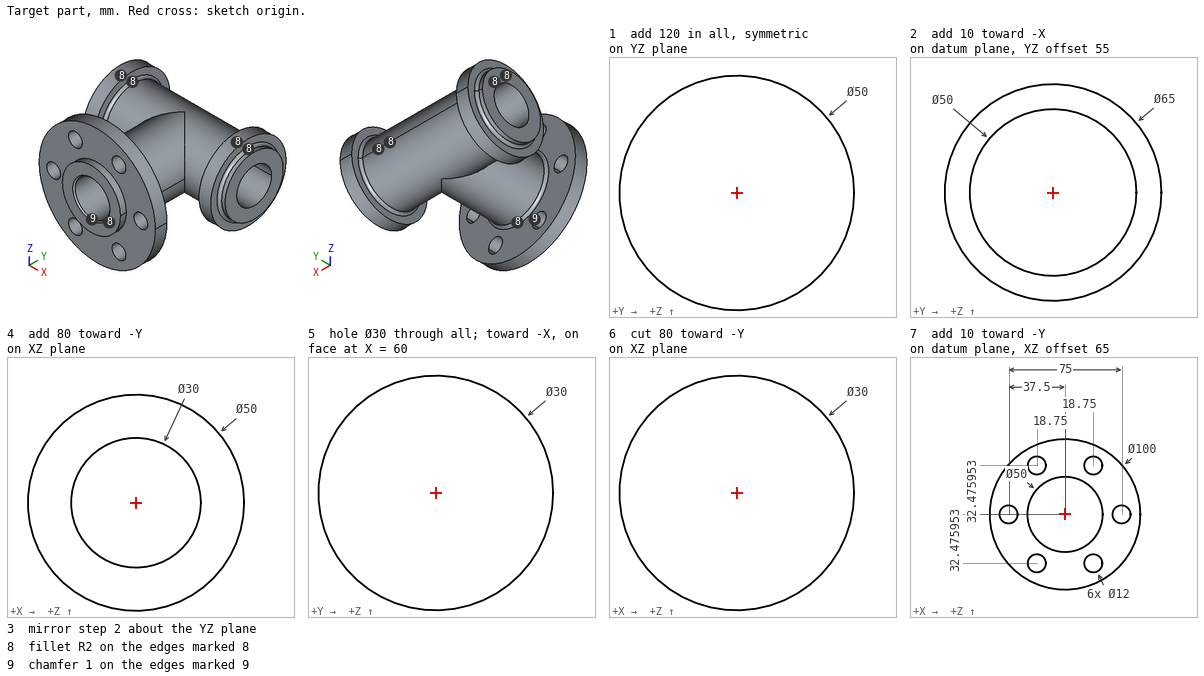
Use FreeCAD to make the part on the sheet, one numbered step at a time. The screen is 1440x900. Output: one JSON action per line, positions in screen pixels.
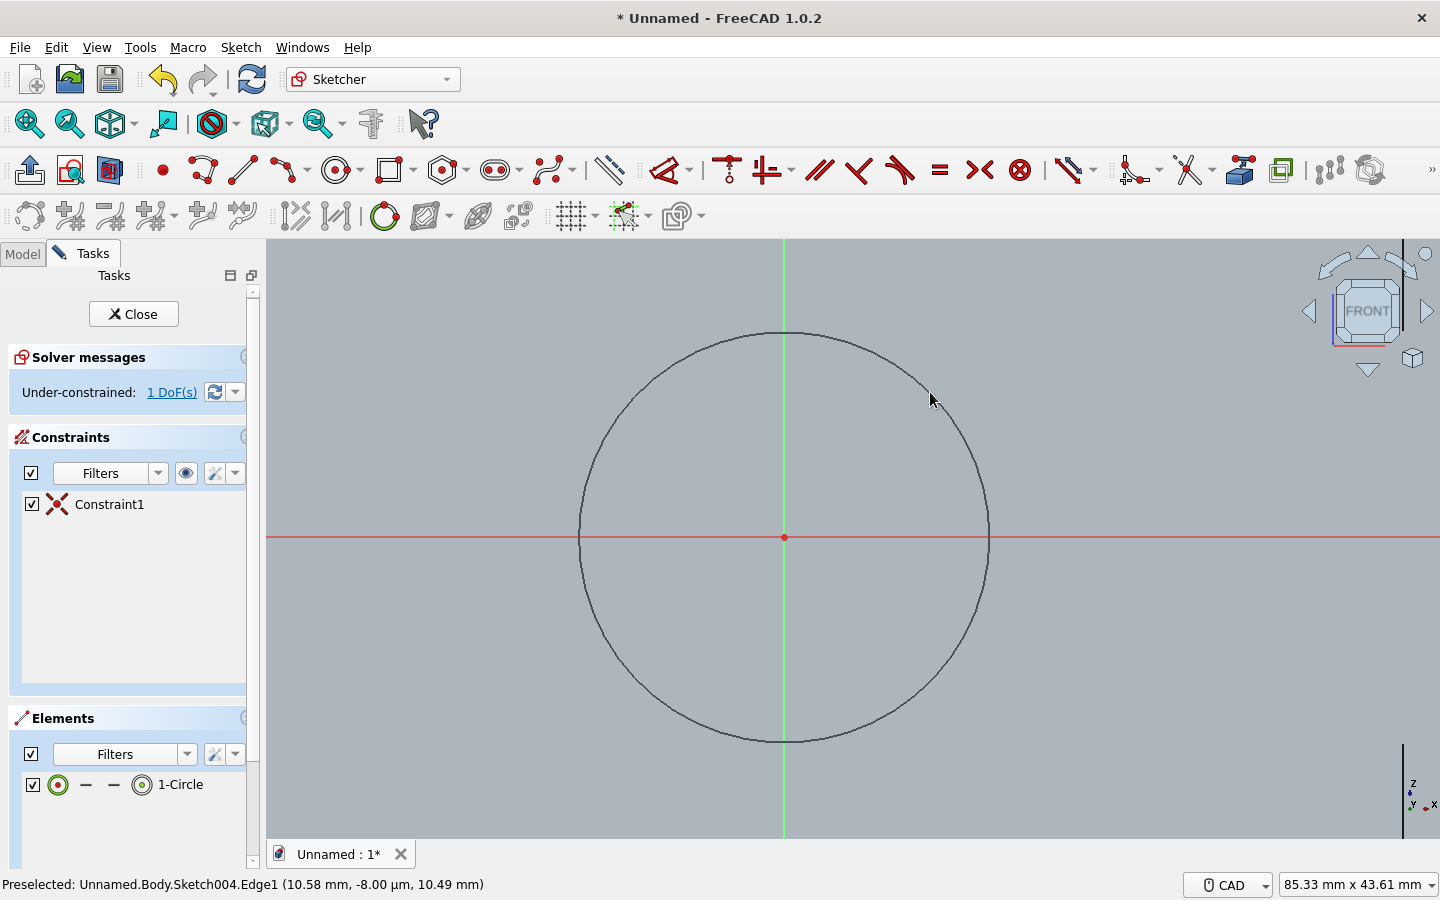
{"action": "left_click", "coordinate": [929, 392]}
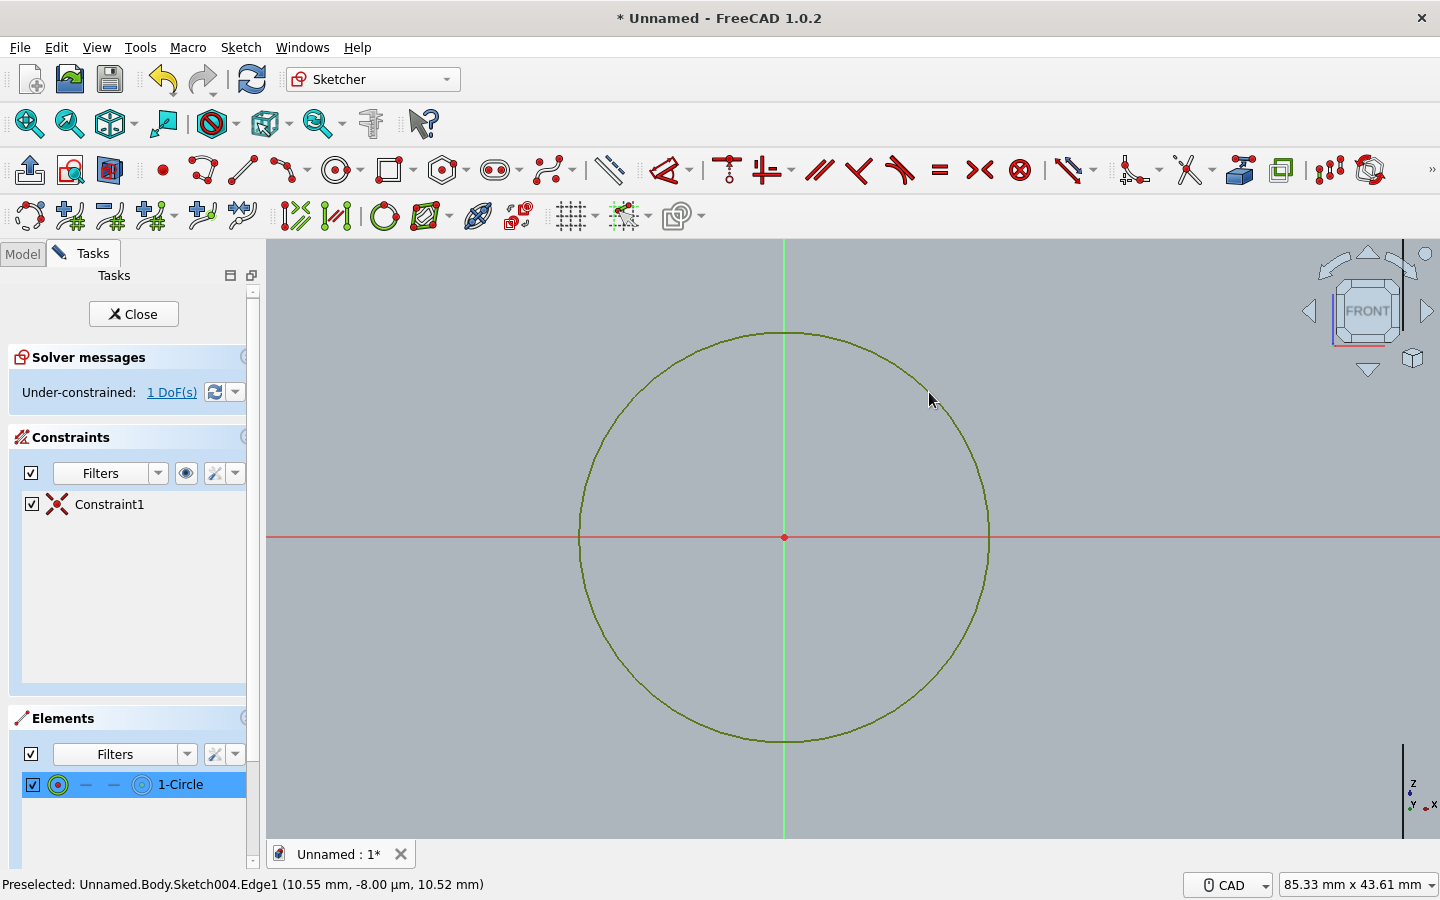
{"action": "key", "text": "k o"}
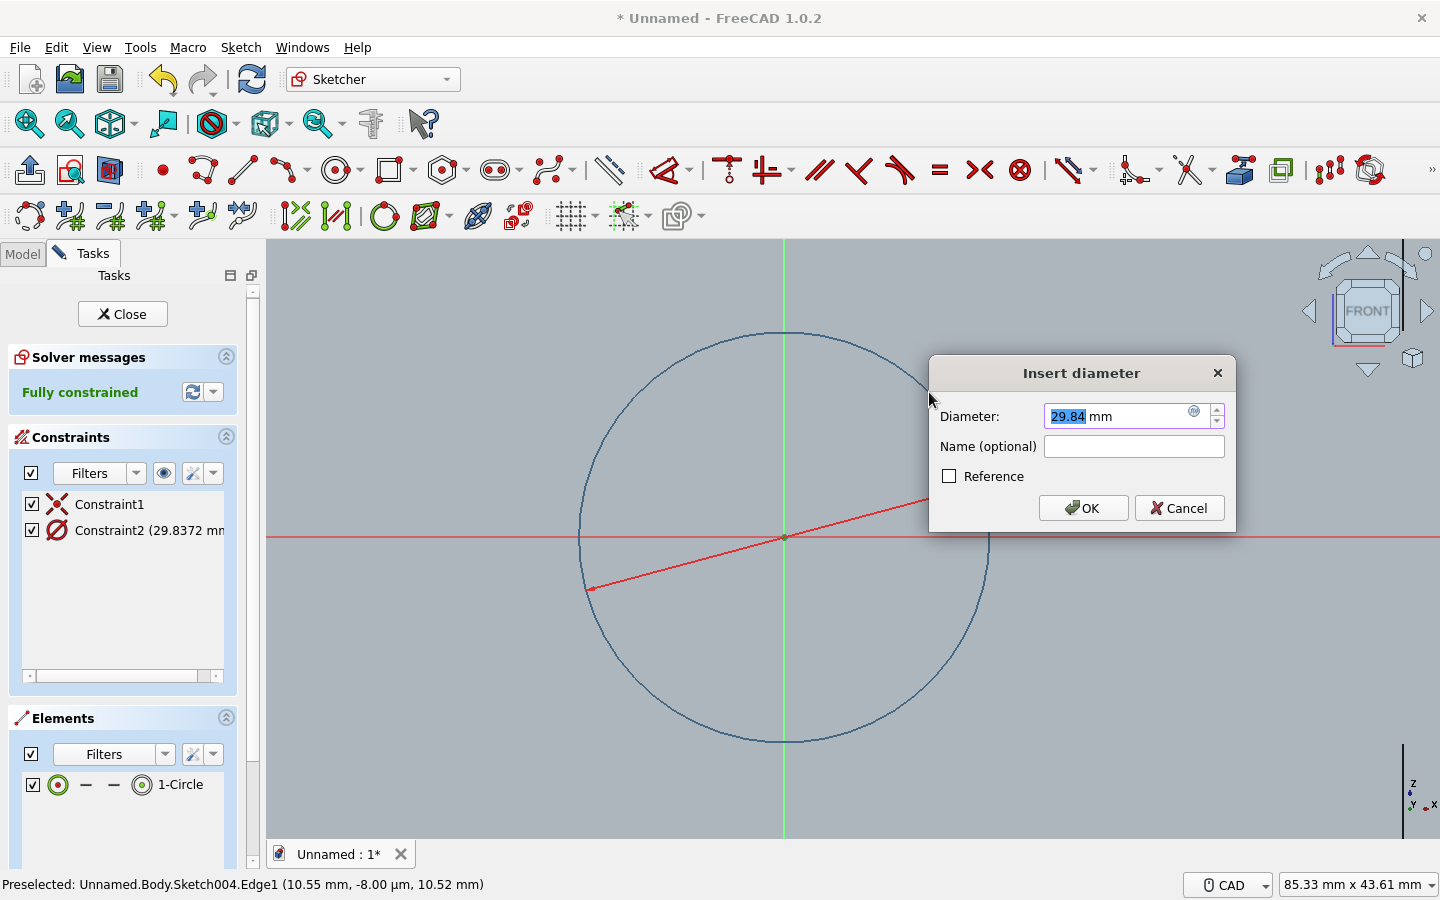
{"action": "type", "text": "30"}
{"action": "key", "text": "Return"}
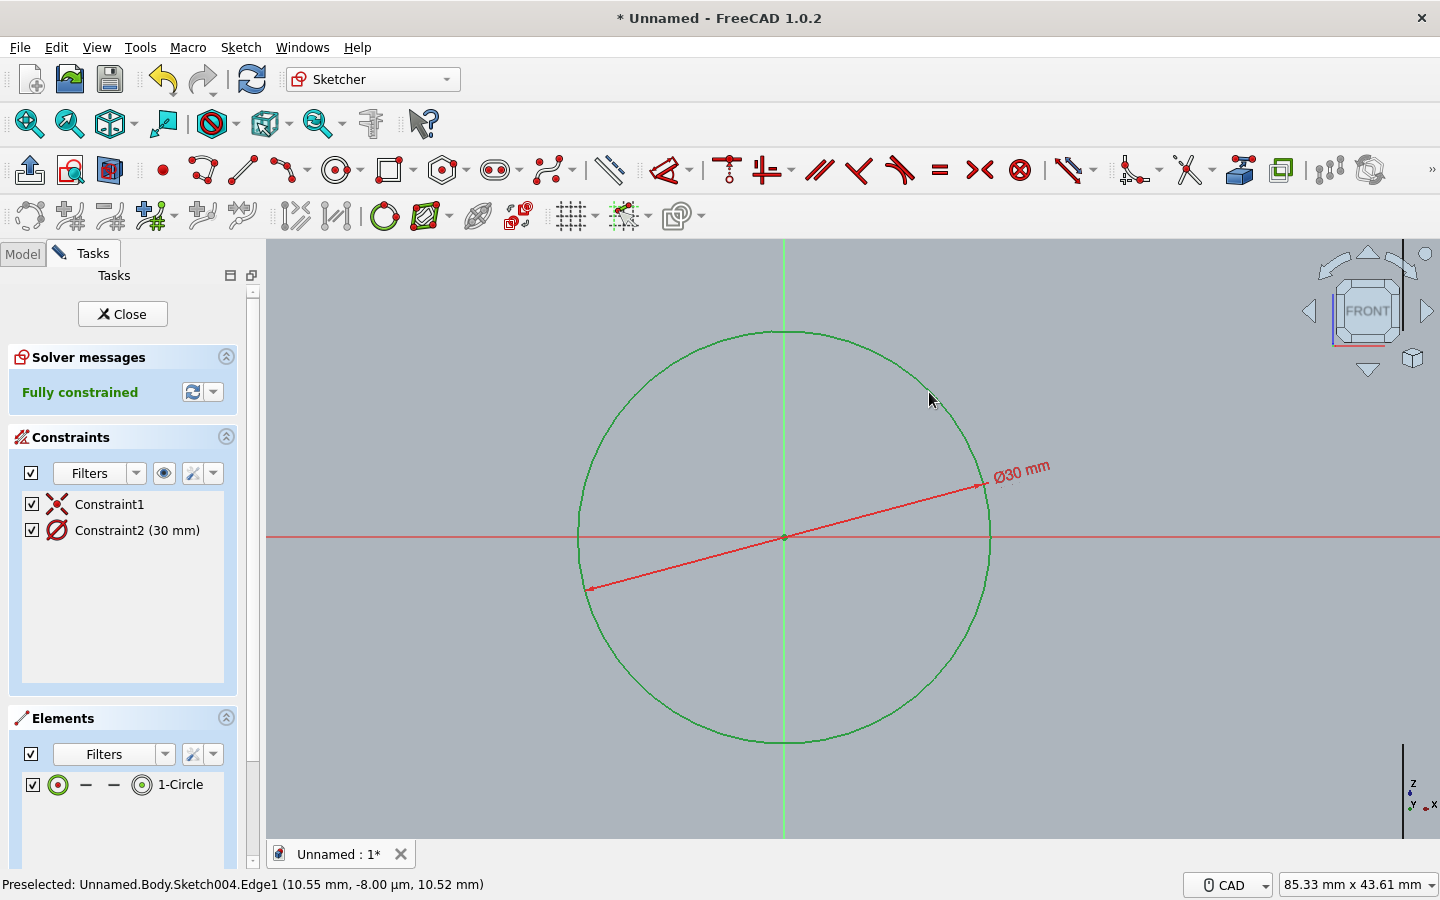
{"action": "left_click", "coordinate": [123, 314]}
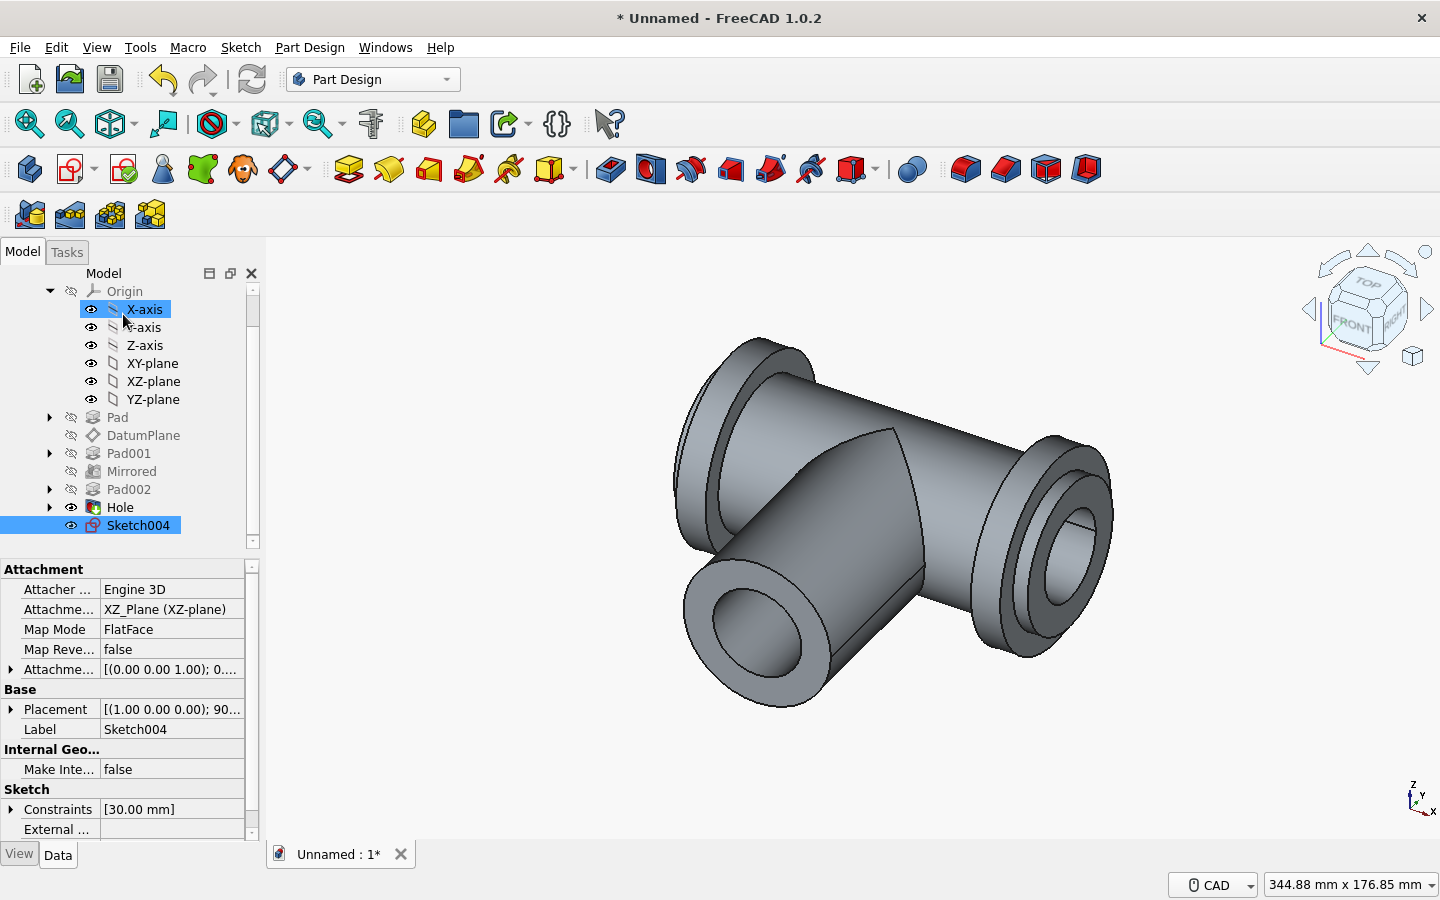
{"action": "left_click", "coordinate": [612, 170]}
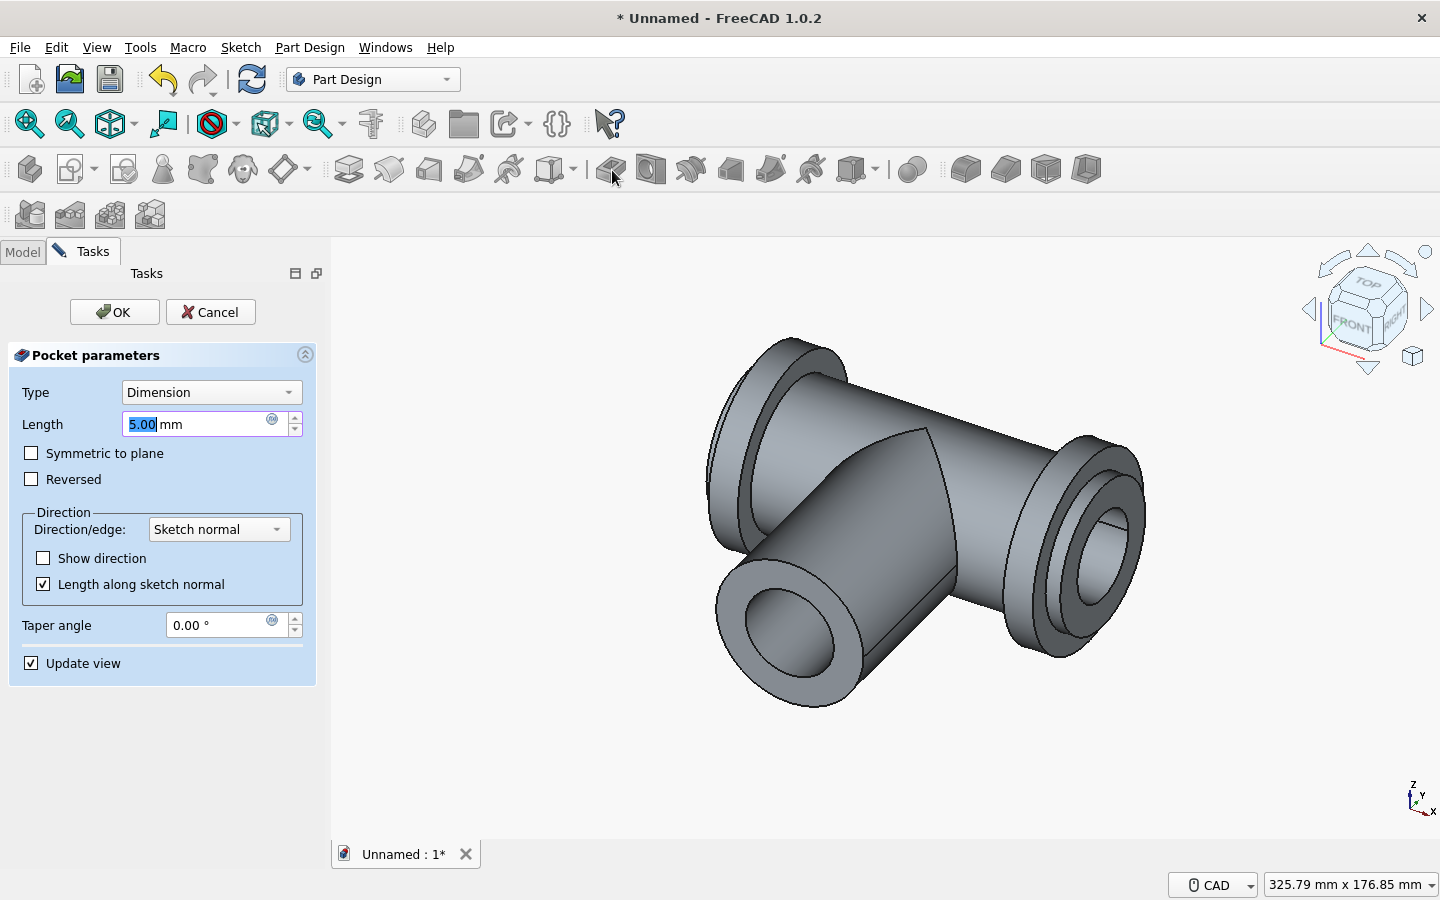
{"action": "type", "text": "80"}
{"action": "key", "text": "Tab"}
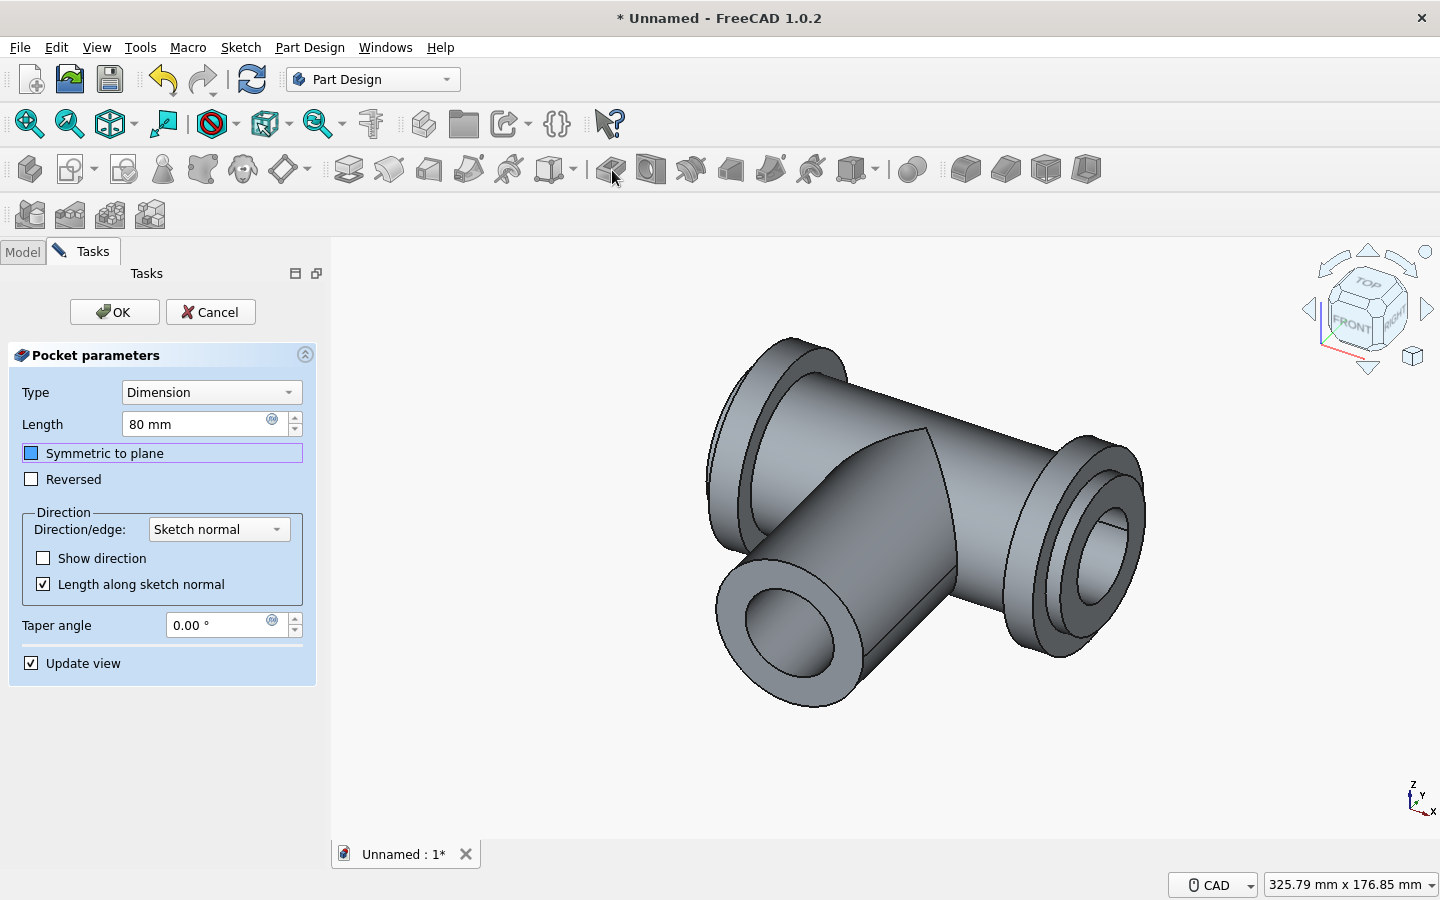
{"action": "left_click", "coordinate": [30, 479]}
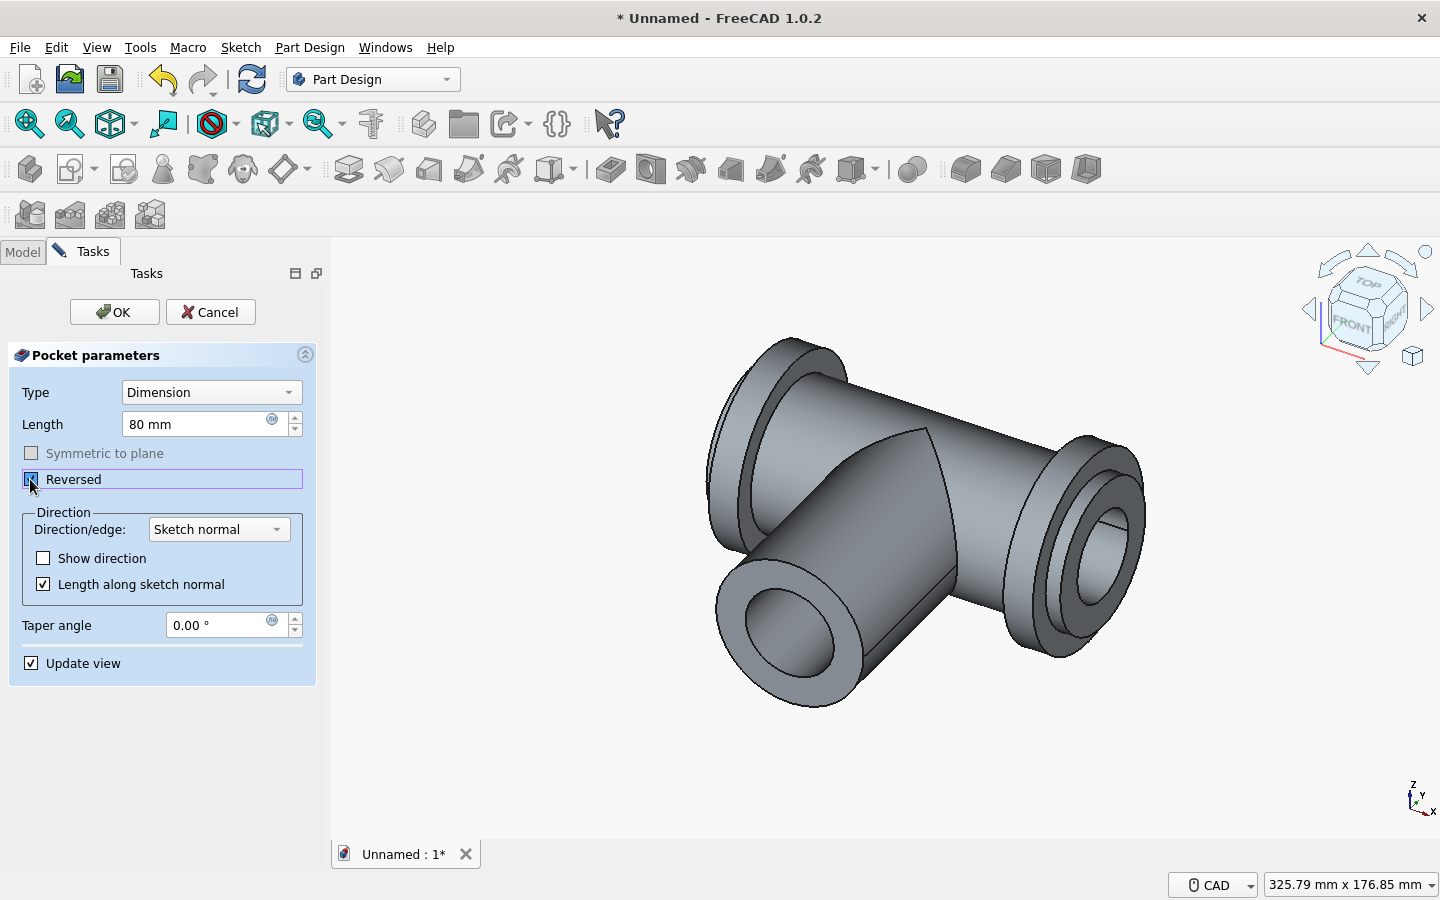
{"action": "left_click", "coordinate": [115, 312]}